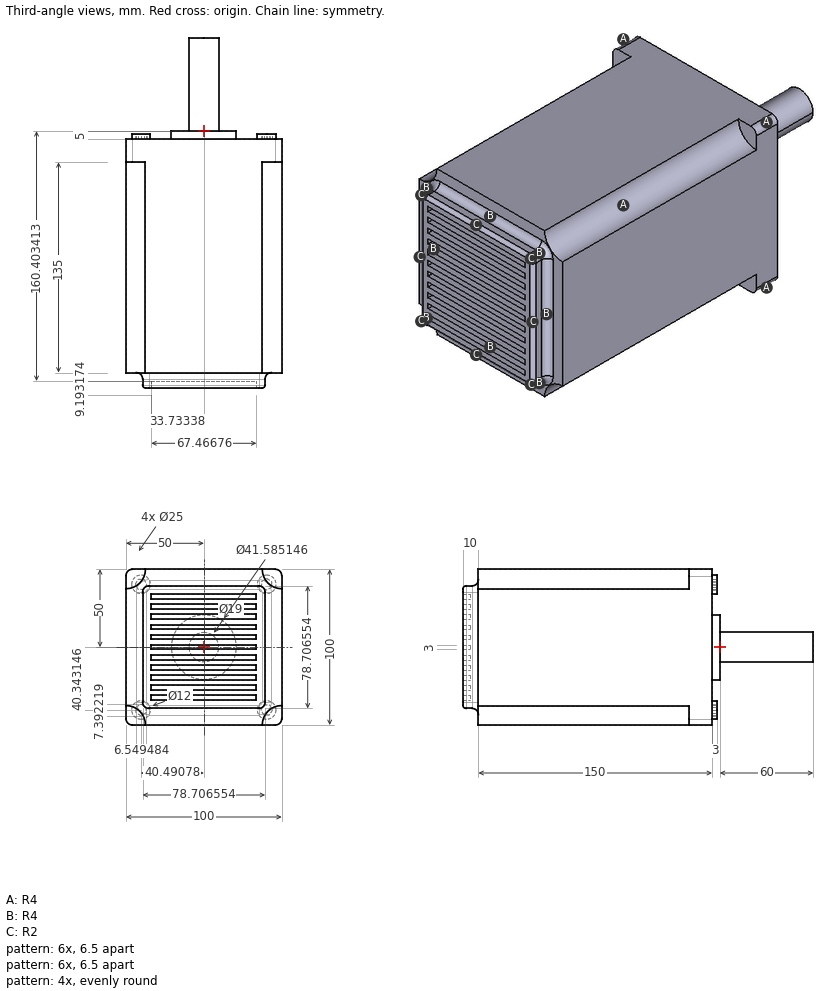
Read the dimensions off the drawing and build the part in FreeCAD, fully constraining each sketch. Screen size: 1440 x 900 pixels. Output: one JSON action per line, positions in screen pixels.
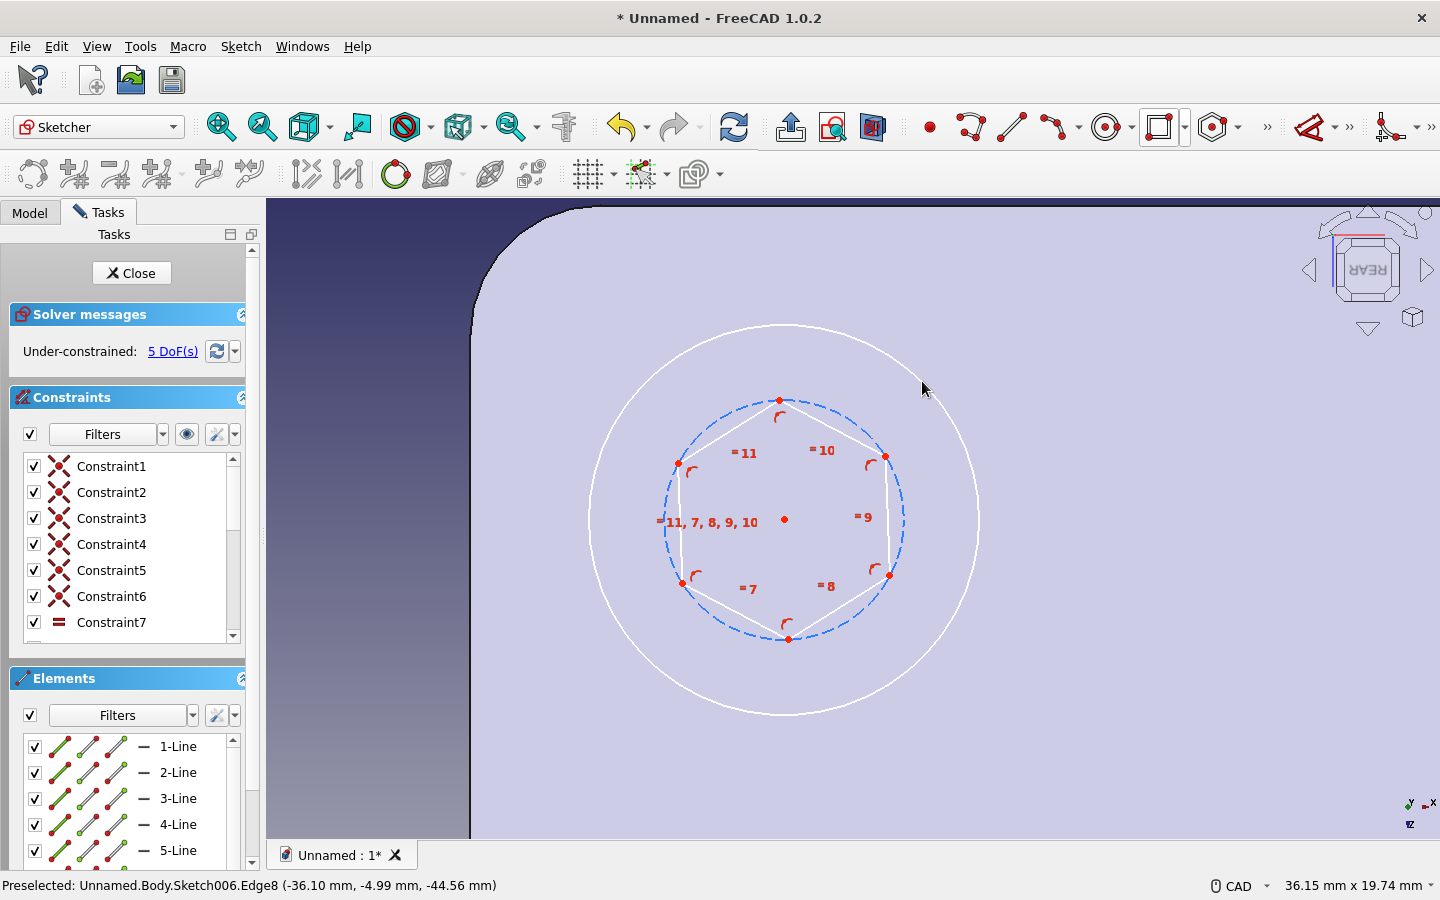
{"action": "left_click", "coordinate": [1308, 128]}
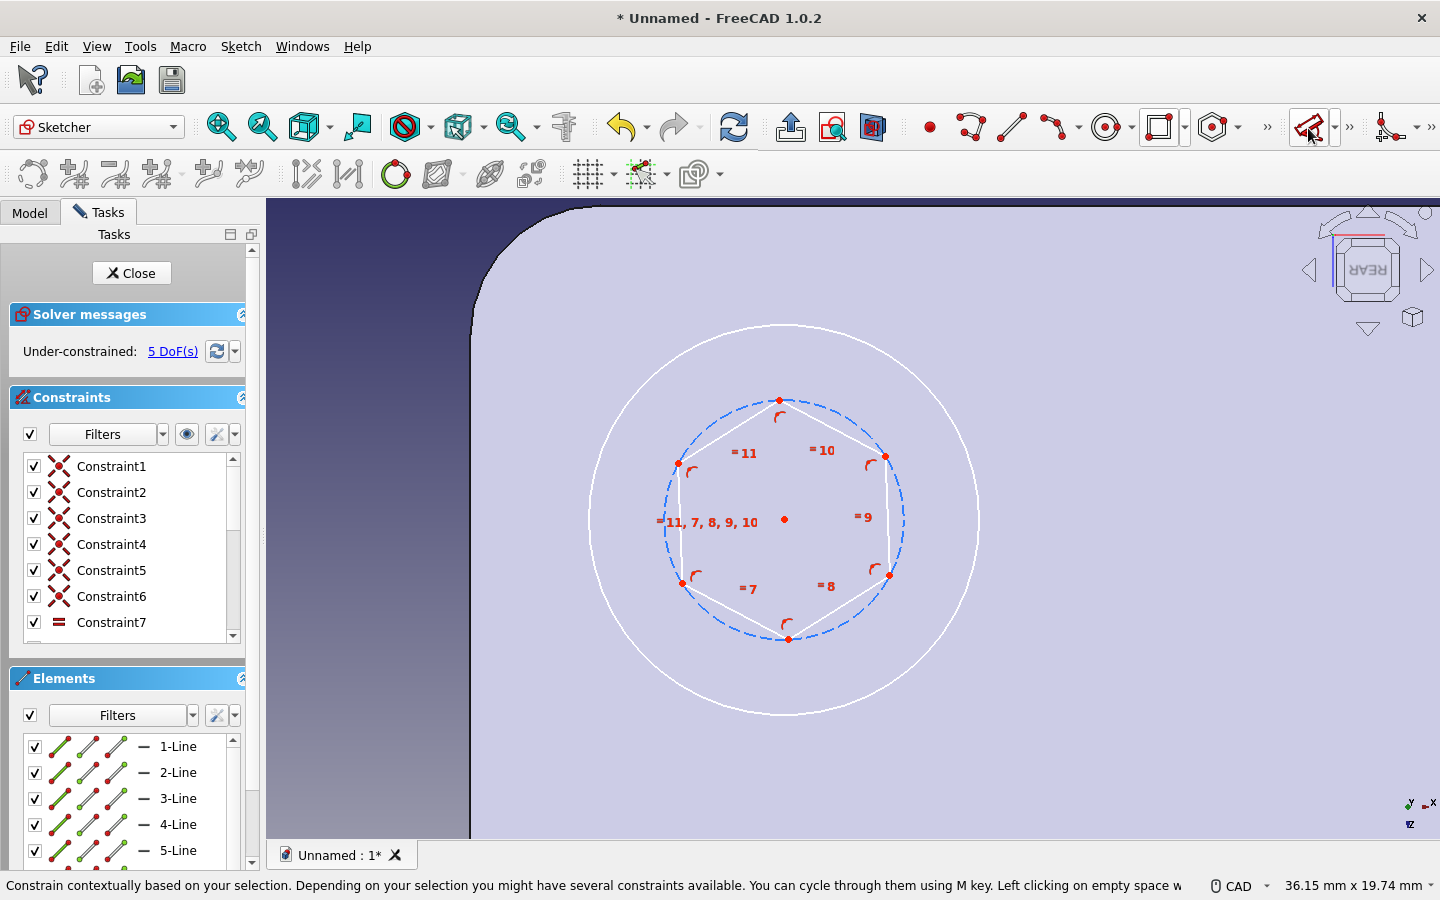
{"action": "left_click", "coordinate": [922, 382]}
{"action": "left_click", "coordinate": [945, 359]}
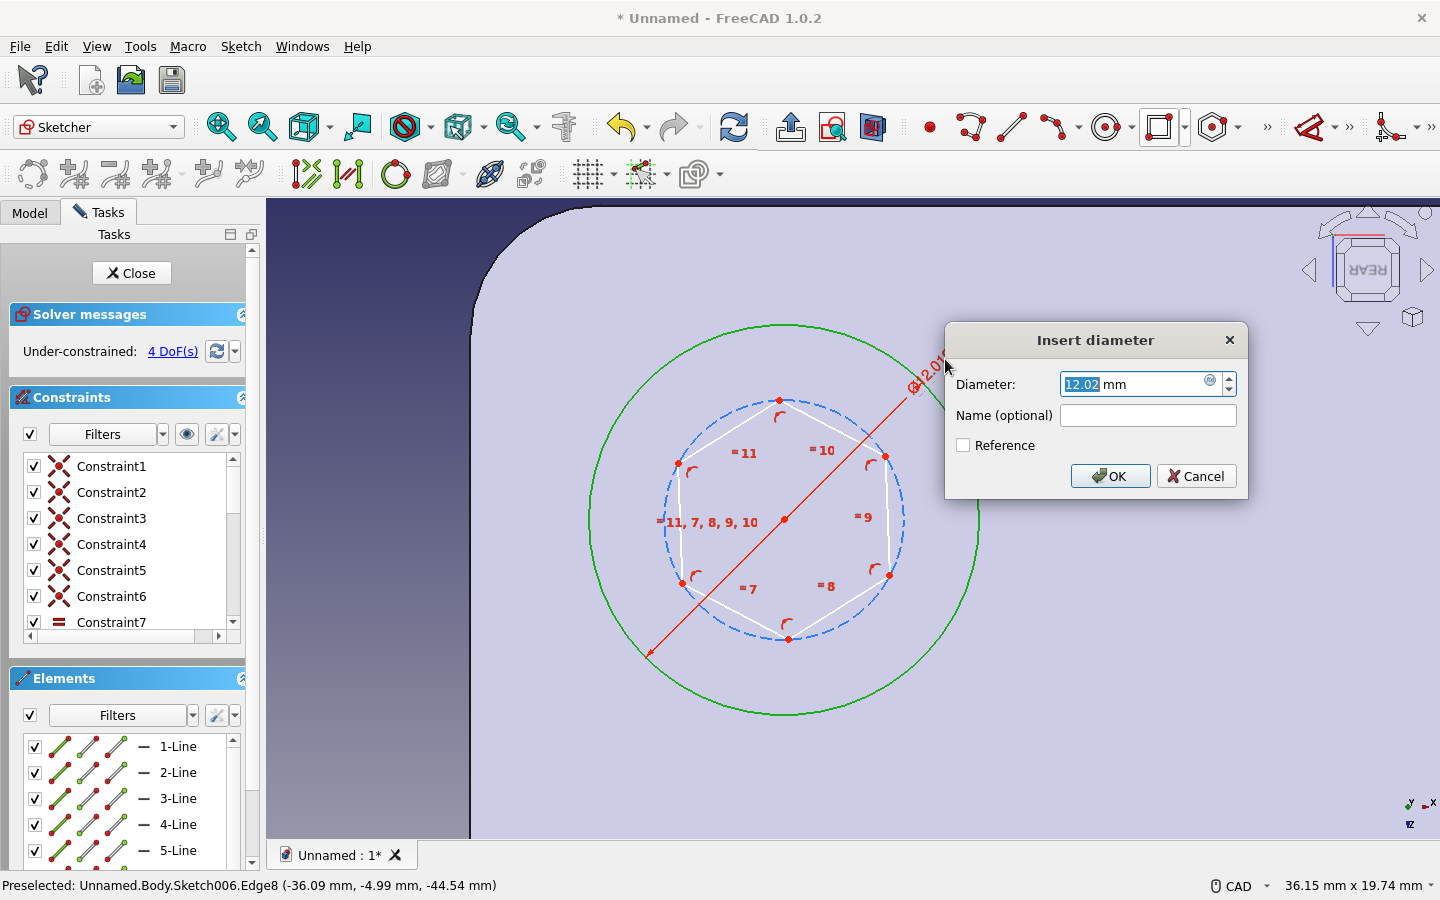
{"action": "type", "text": "12"}
{"action": "key", "text": "Return"}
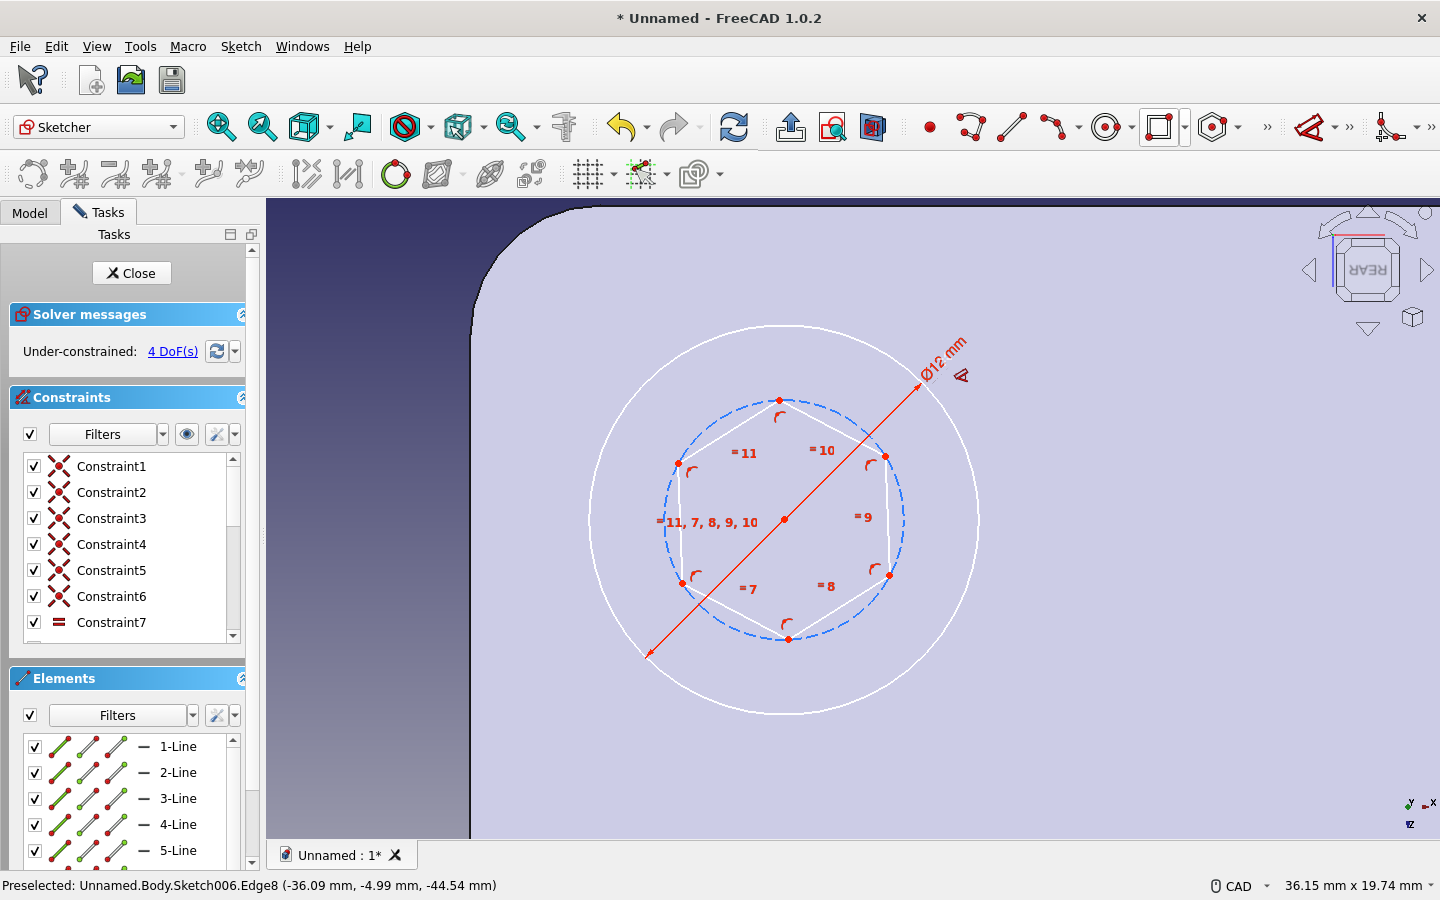
{"action": "left_click", "coordinate": [678, 464]}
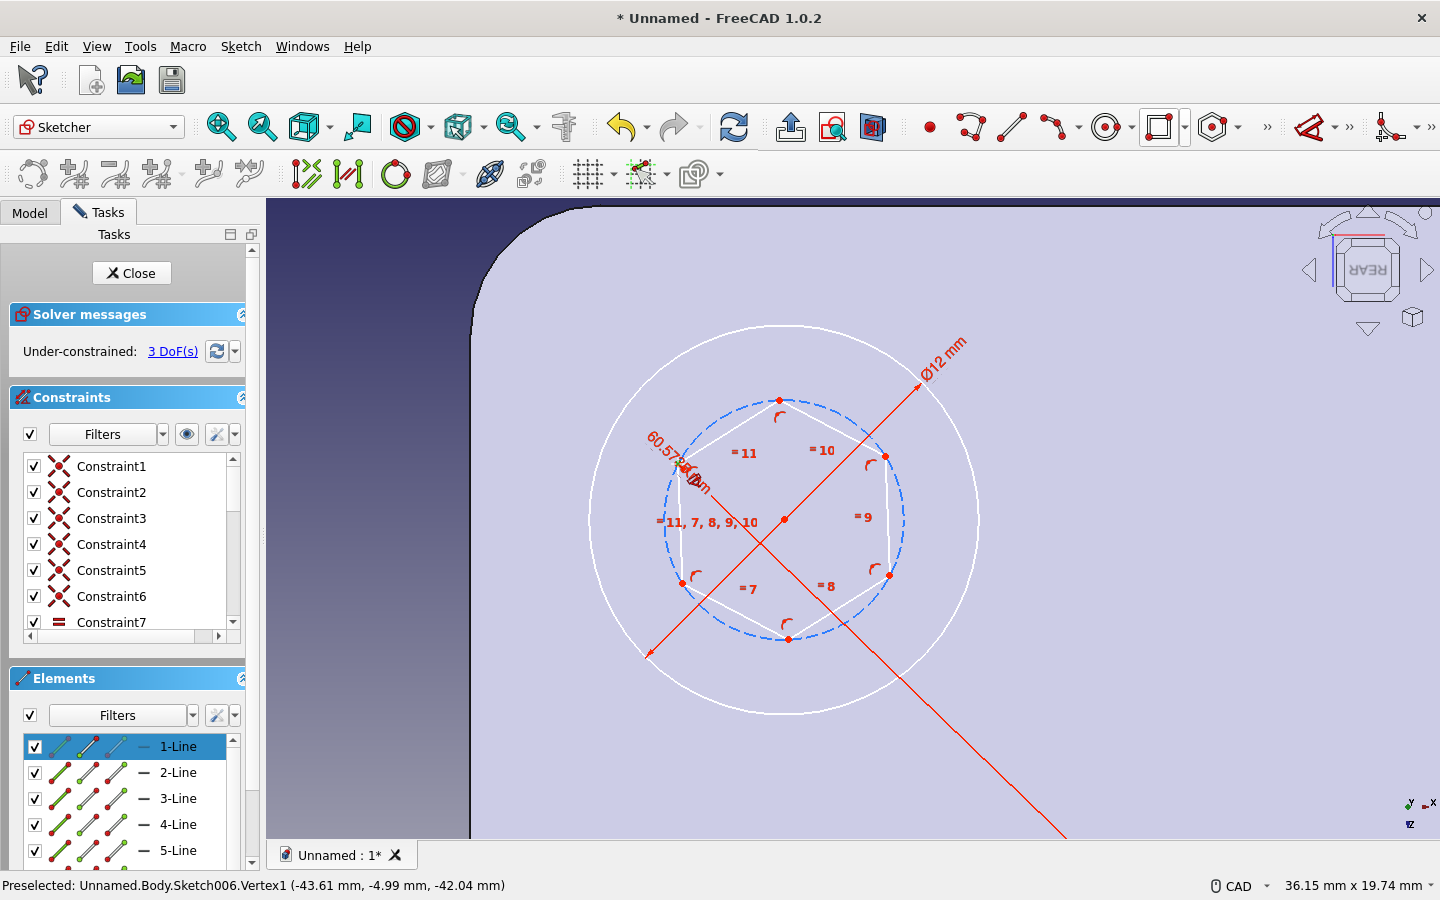
{"action": "left_click", "coordinate": [890, 576]}
{"action": "left_click", "coordinate": [784, 610]}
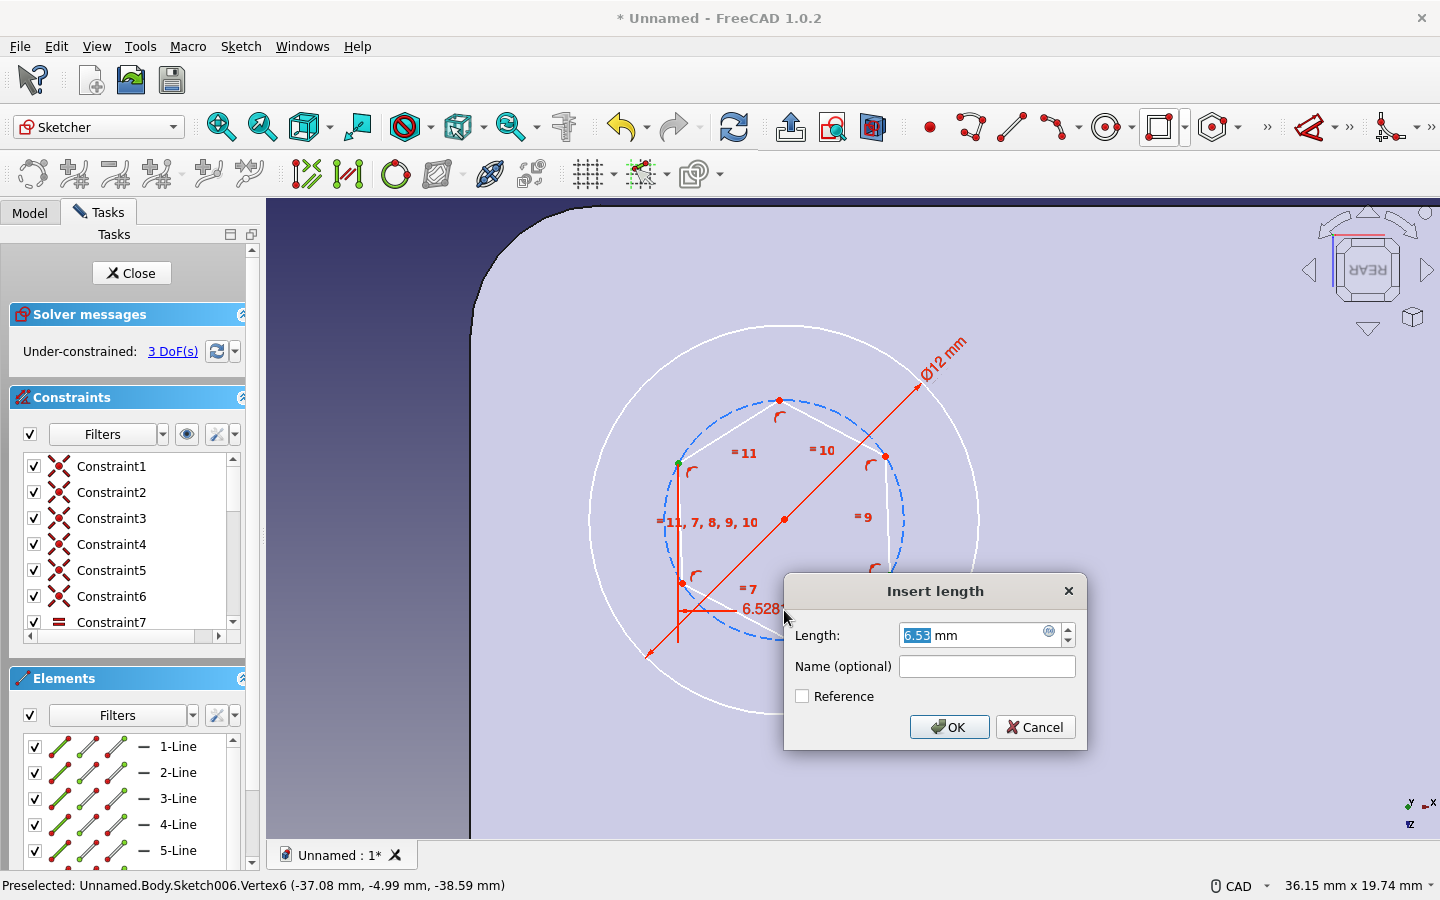
{"action": "type", "text": "6.549484"}
{"action": "key", "text": "Return"}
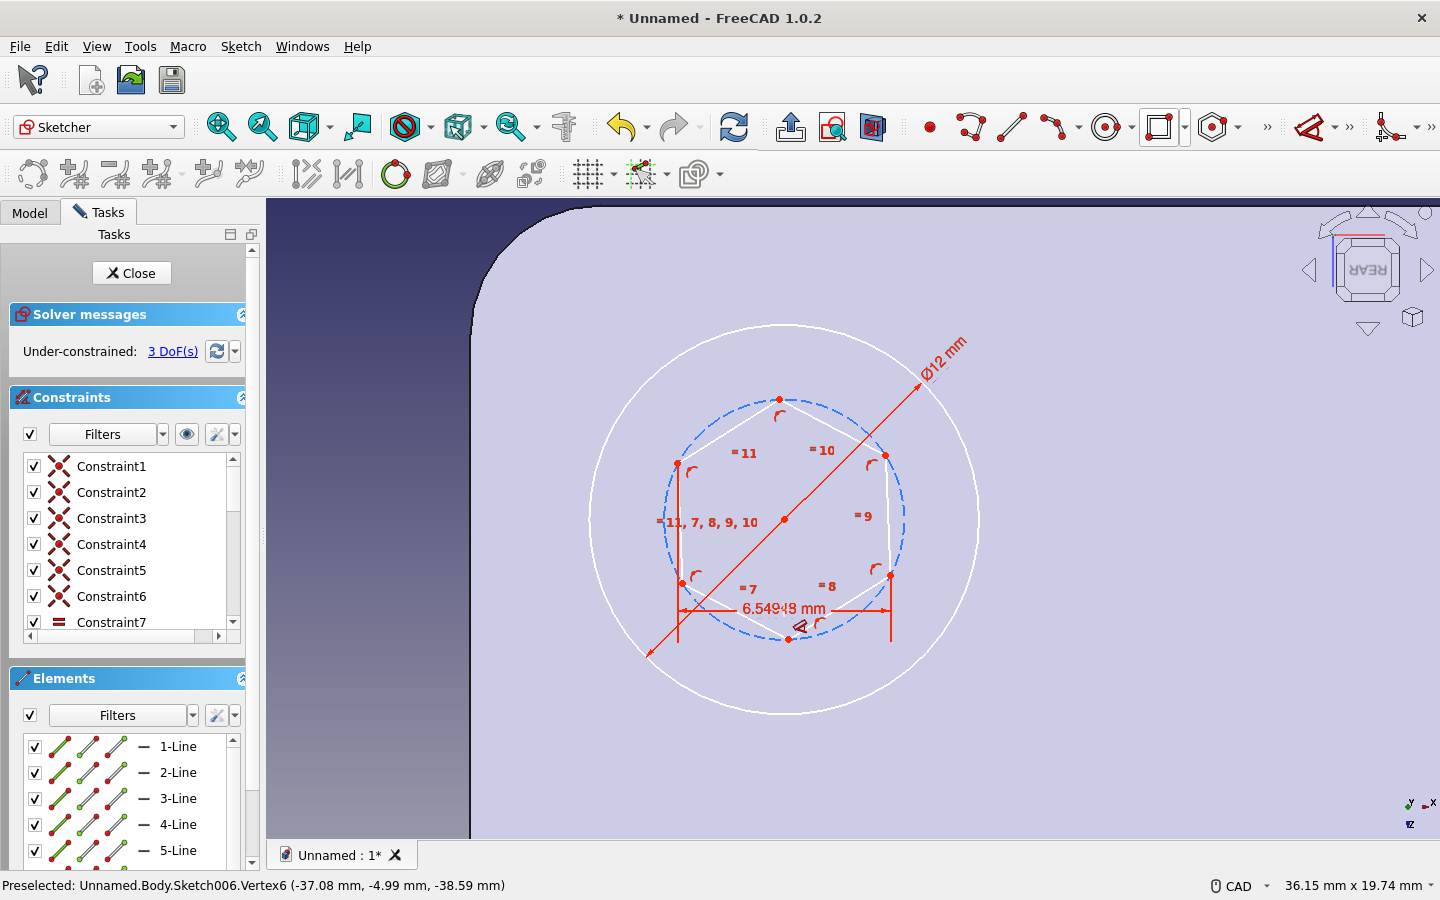
{"action": "left_click", "coordinate": [789, 640]}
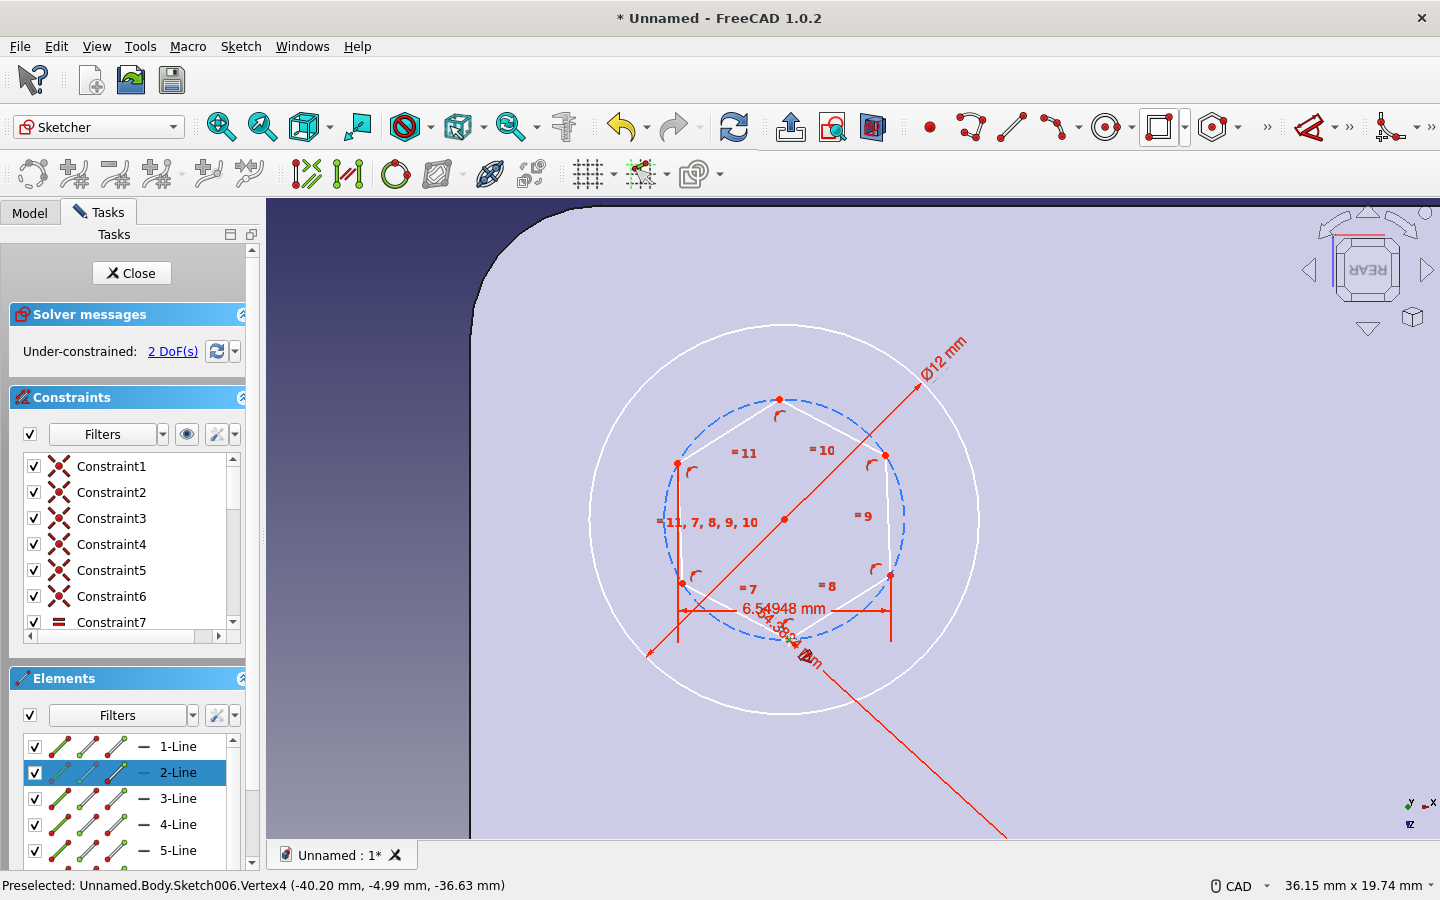
{"action": "left_click", "coordinate": [779, 400]}
{"action": "left_click", "coordinate": [823, 520]}